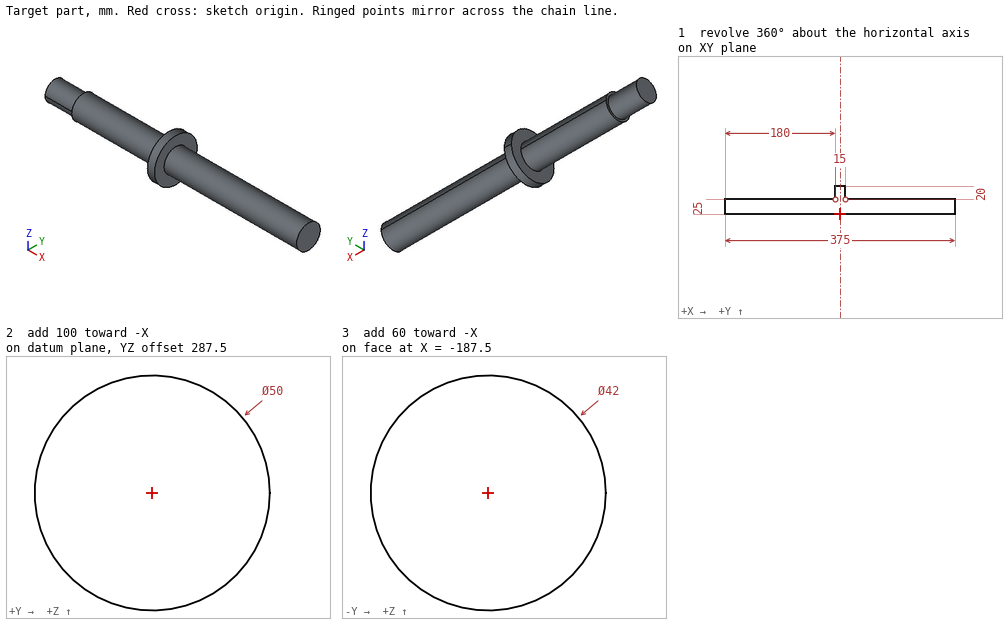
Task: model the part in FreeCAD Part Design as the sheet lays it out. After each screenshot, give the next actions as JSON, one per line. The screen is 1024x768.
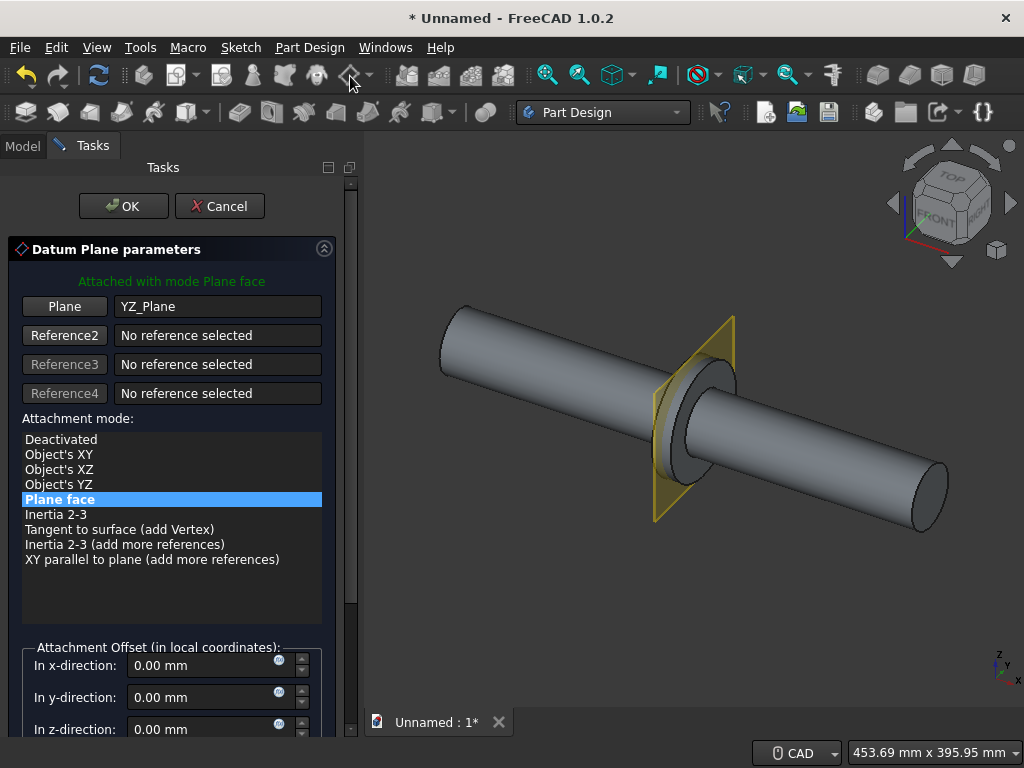
{"action": "scroll", "coordinate": [351, 456], "scroll_direction": "down", "scroll_amount": 2}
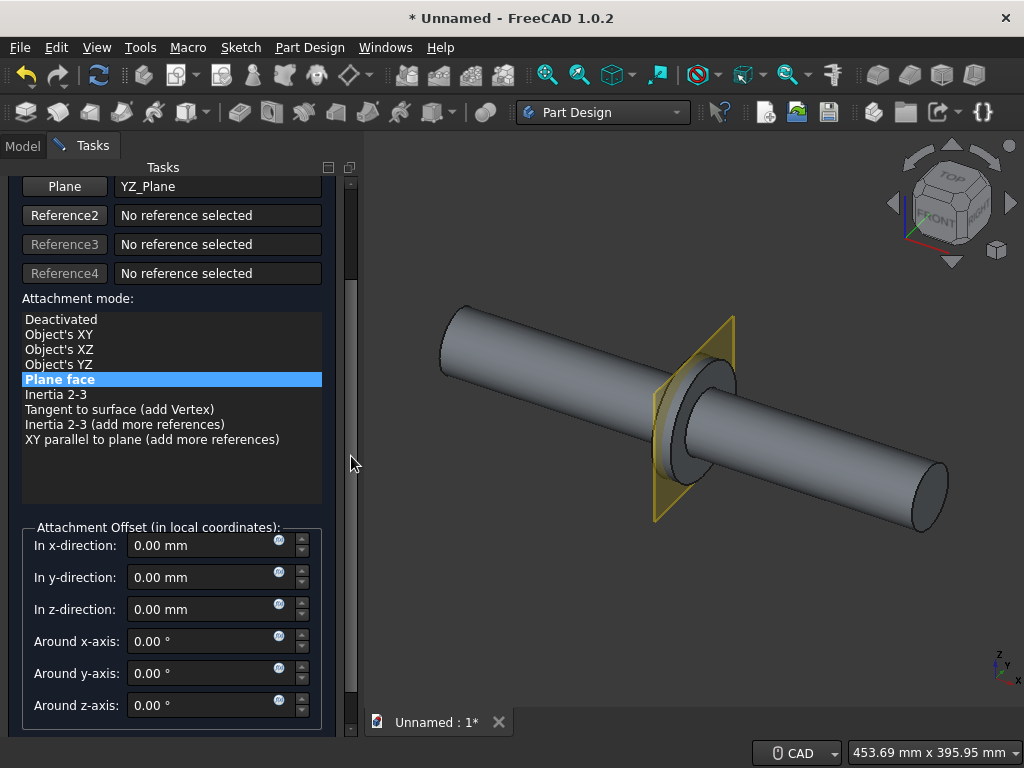
{"action": "triple_click", "coordinate": [210, 609]}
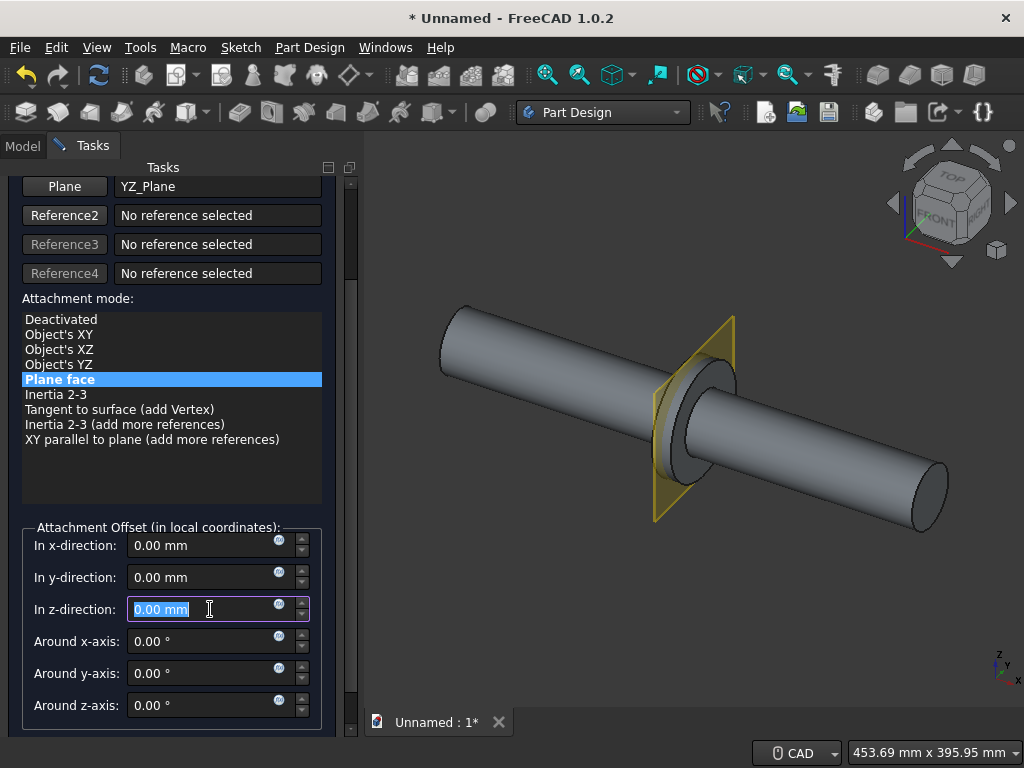
{"action": "type", "text": "287.5"}
{"action": "key", "text": "Tab"}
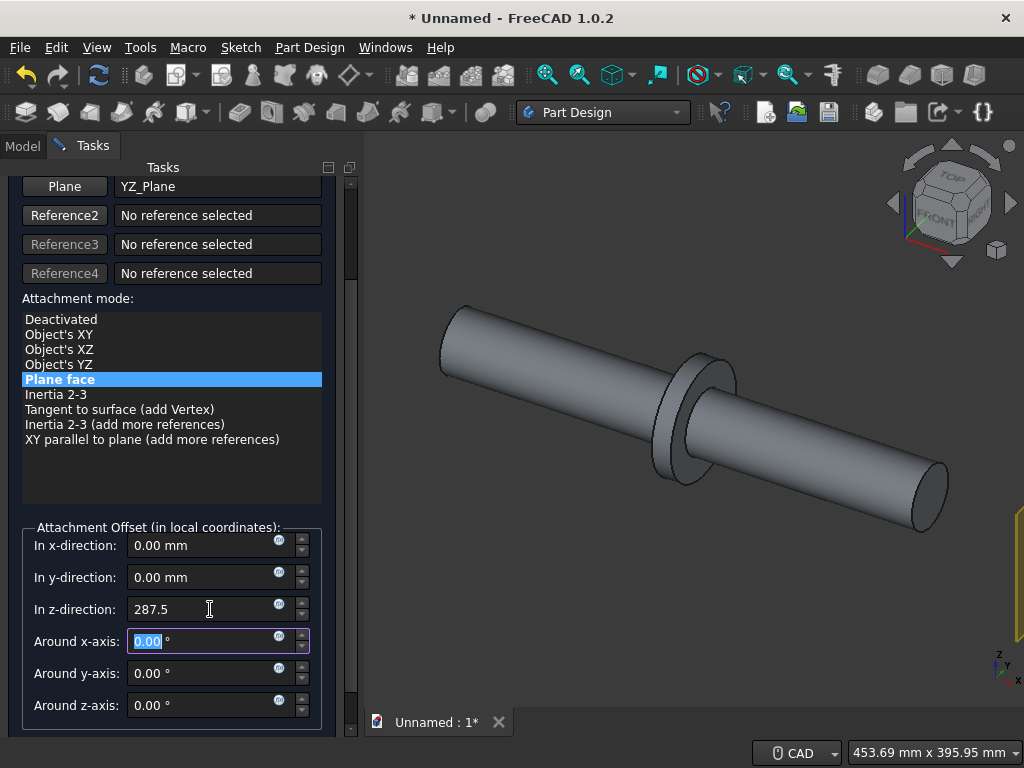
{"action": "scroll", "coordinate": [351, 456], "scroll_direction": "up", "scroll_amount": 3}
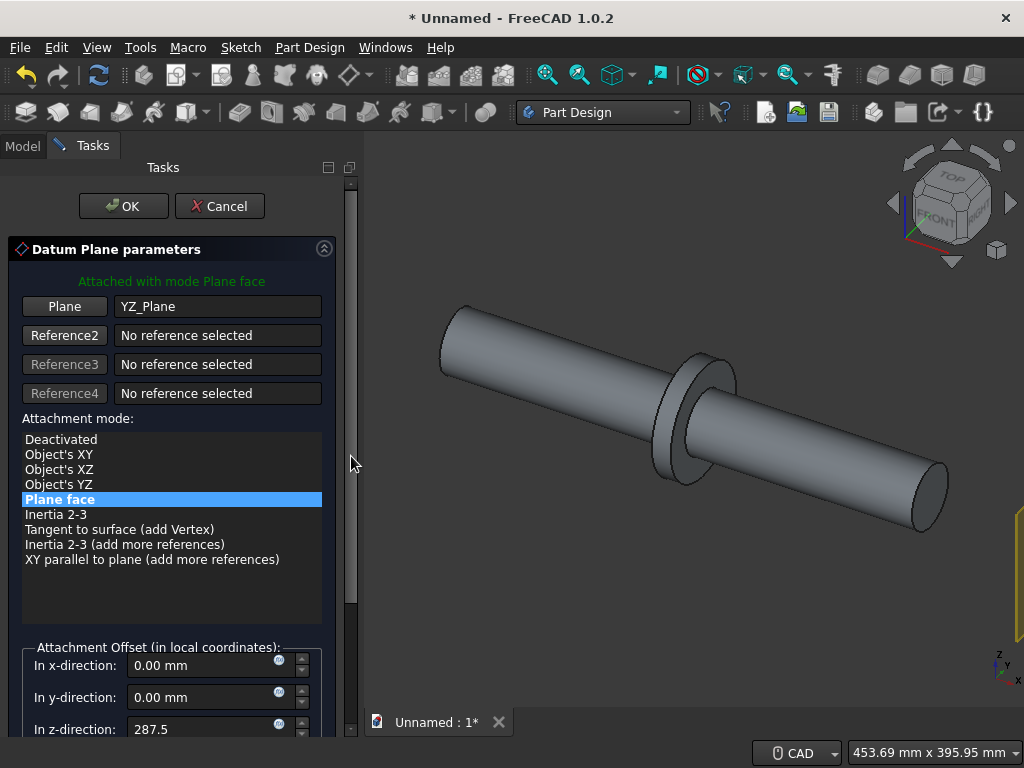
{"action": "left_click", "coordinate": [124, 206]}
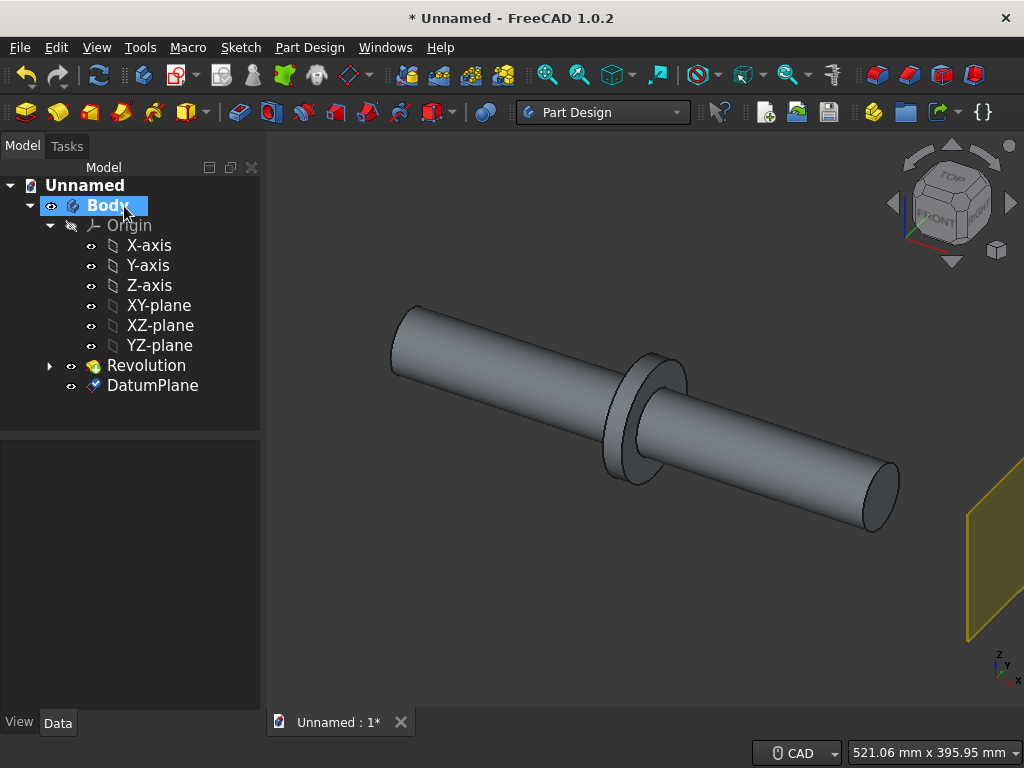
{"action": "left_click", "coordinate": [116, 386]}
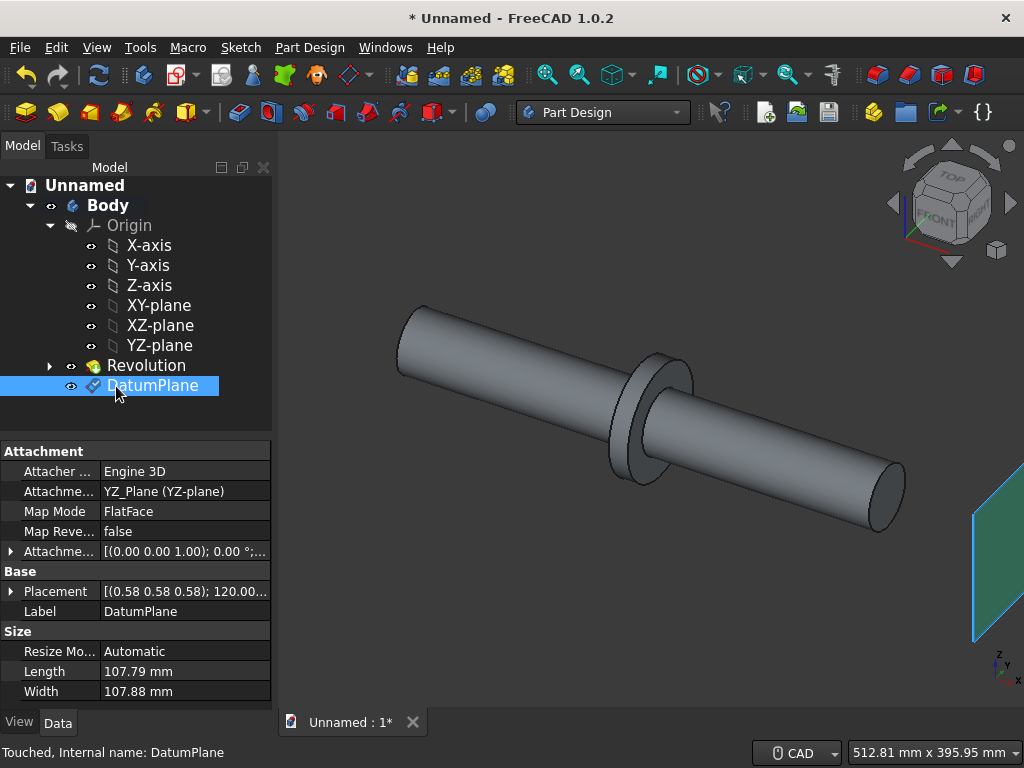
{"action": "left_click", "coordinate": [176, 76]}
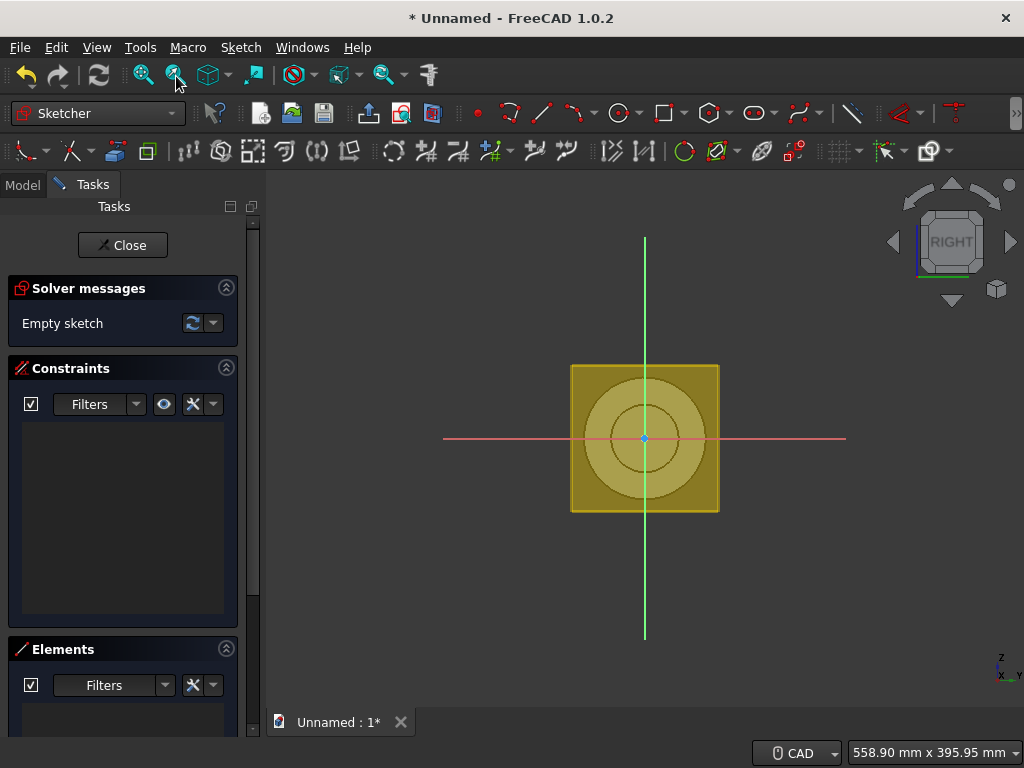
{"action": "scroll", "coordinate": [662, 438], "scroll_direction": "up", "scroll_amount": 8}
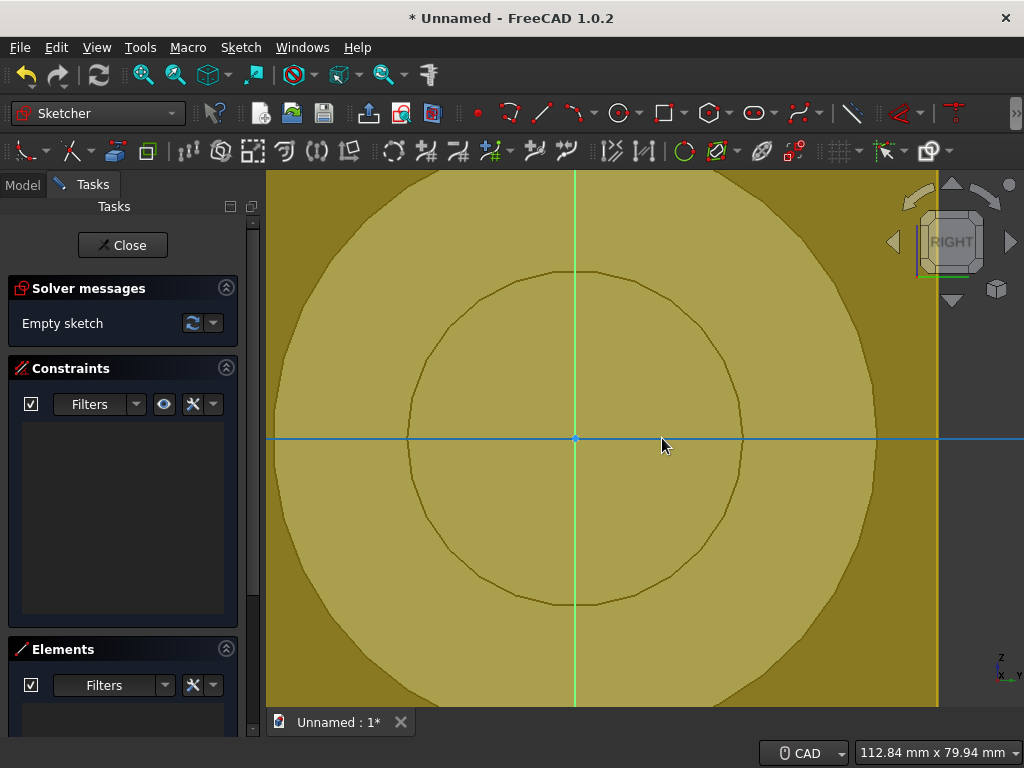
{"action": "left_click", "coordinate": [620, 114]}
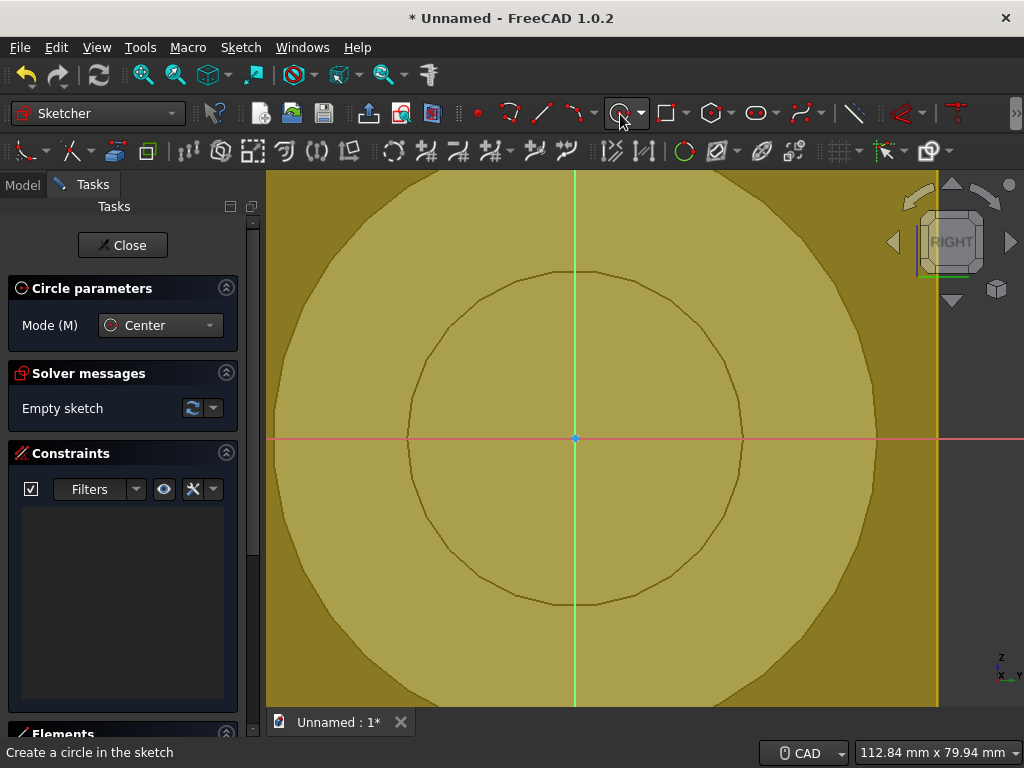
{"action": "left_click", "coordinate": [575, 438]}
{"action": "mouse_move", "coordinate": [694, 320]}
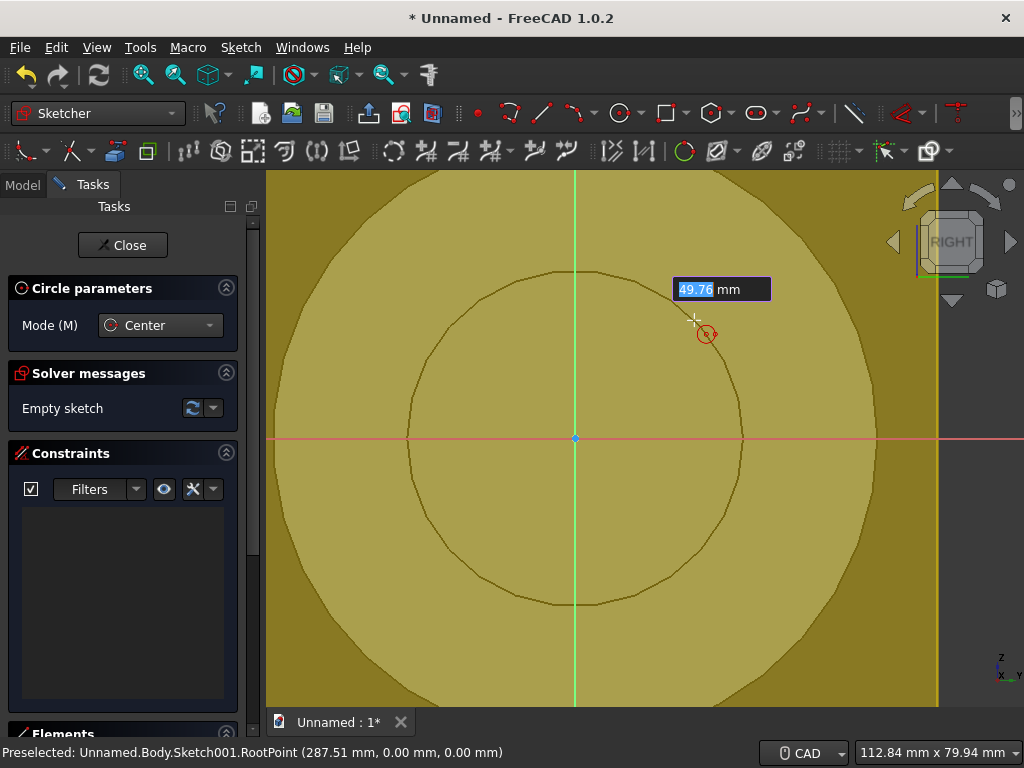
{"action": "type", "text": "50"}
{"action": "key", "text": "Return"}
{"action": "key", "text": "Escape"}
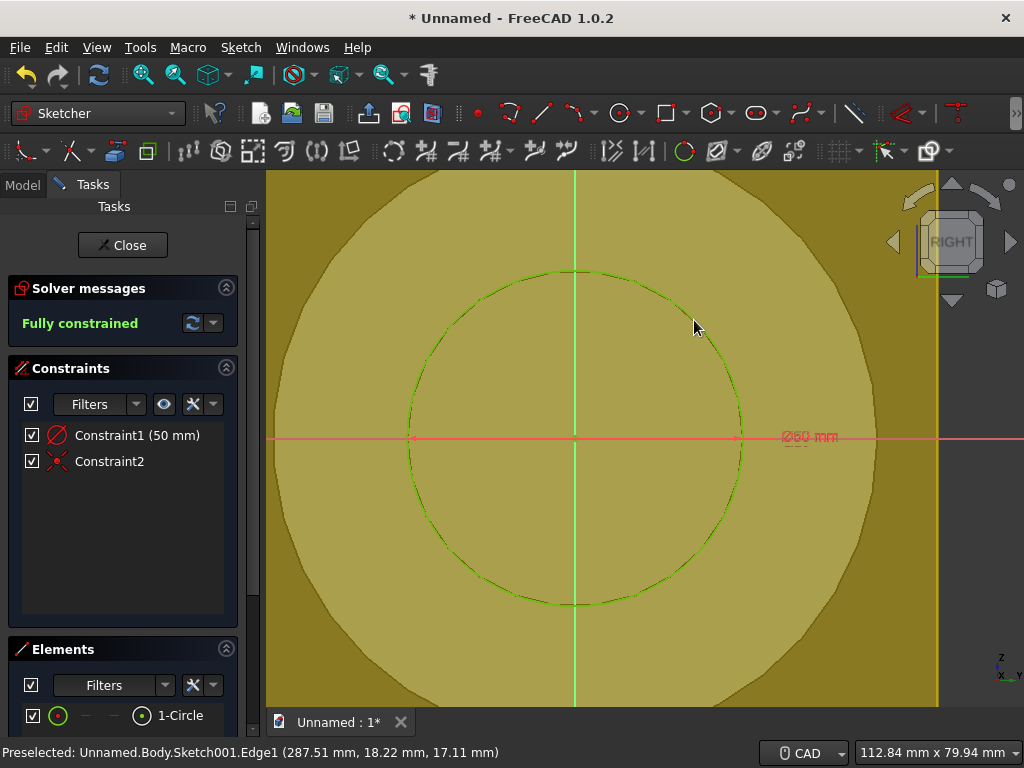
{"action": "left_click", "coordinate": [123, 245]}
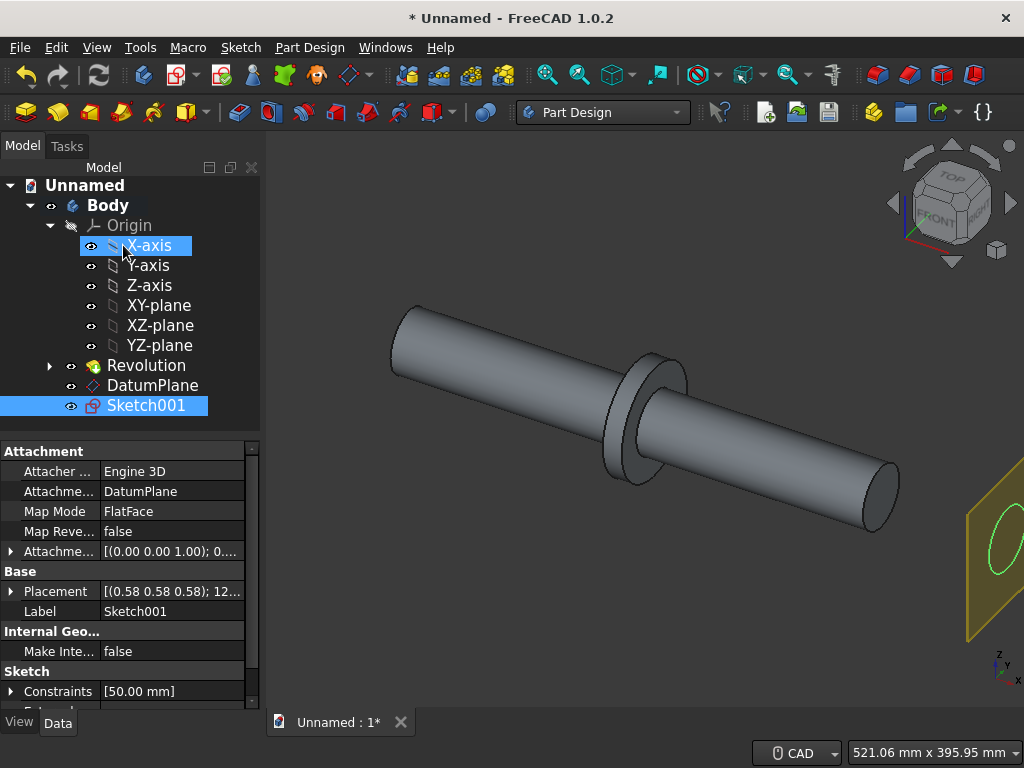
{"action": "left_click", "coordinate": [26, 112]}